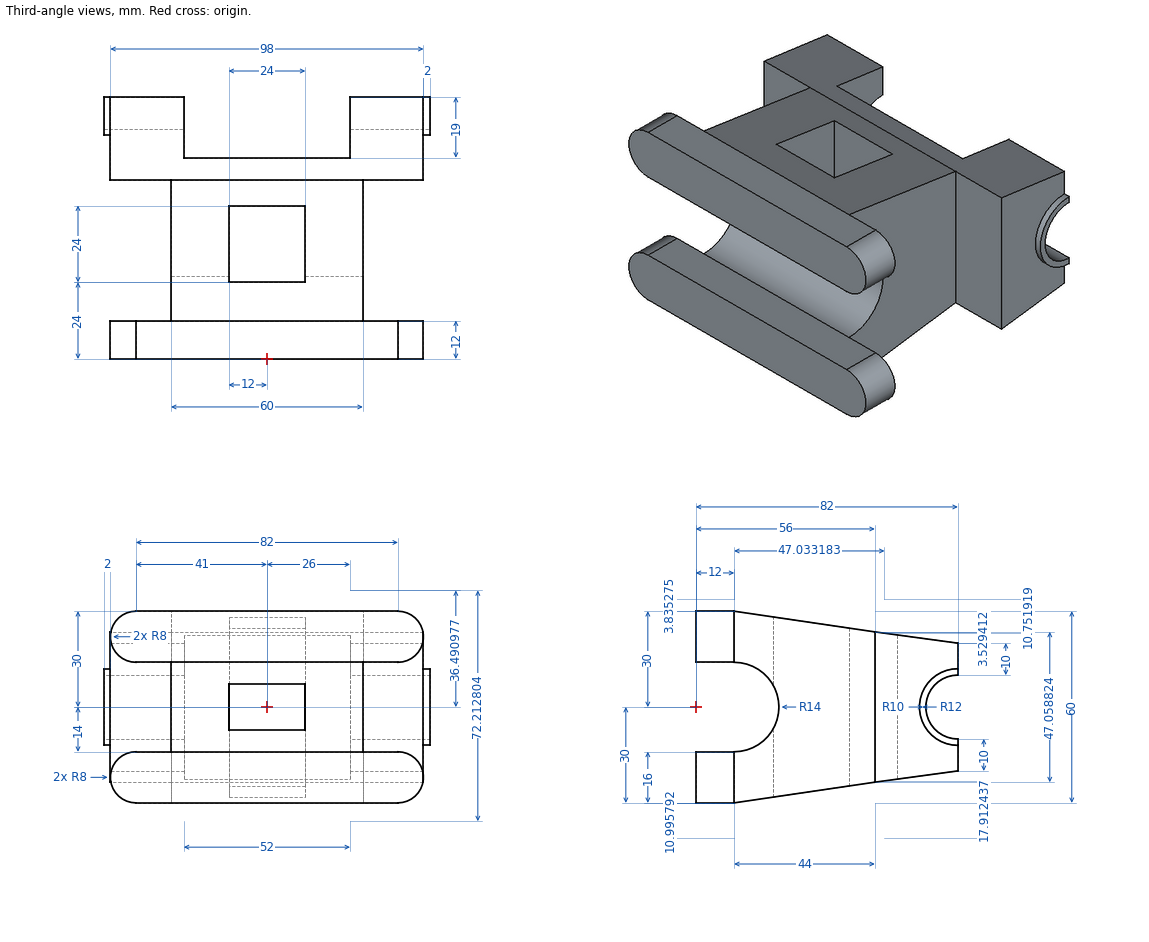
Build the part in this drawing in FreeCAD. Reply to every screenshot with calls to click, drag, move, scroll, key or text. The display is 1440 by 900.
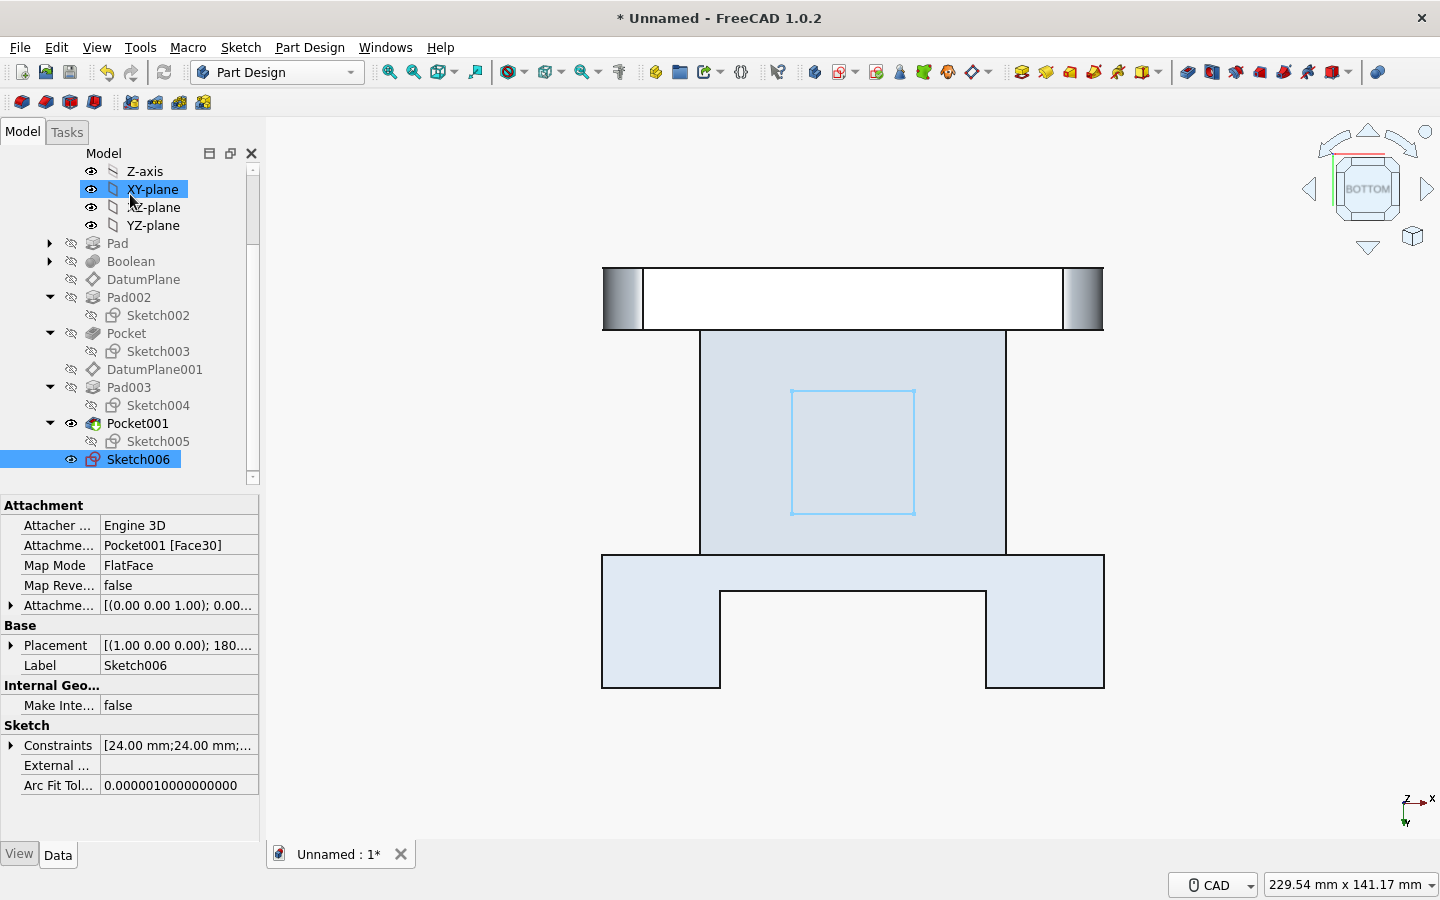
click(1188, 72)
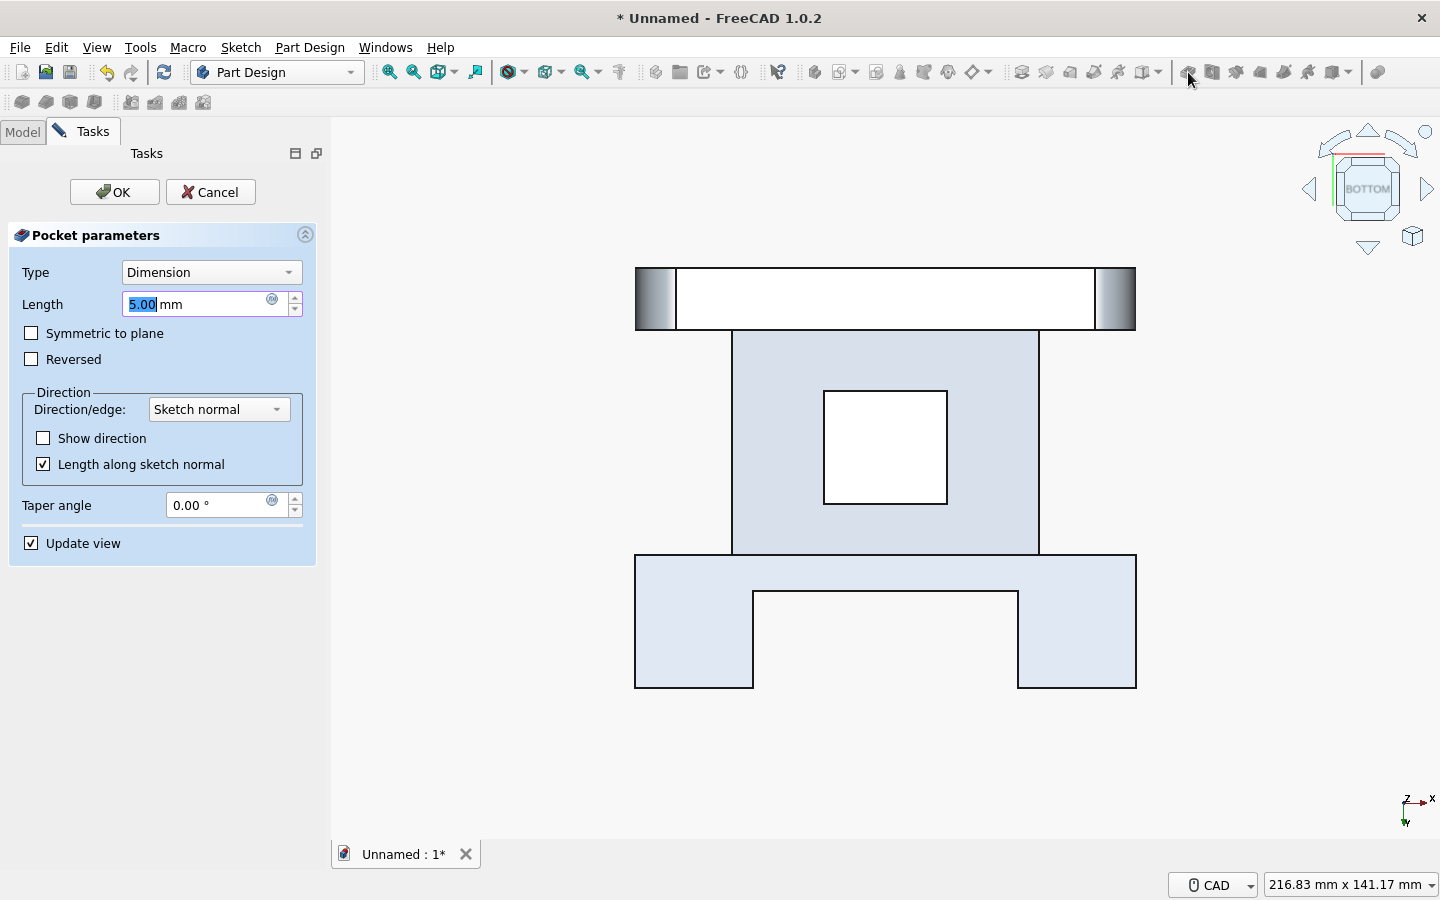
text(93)
key(Tab)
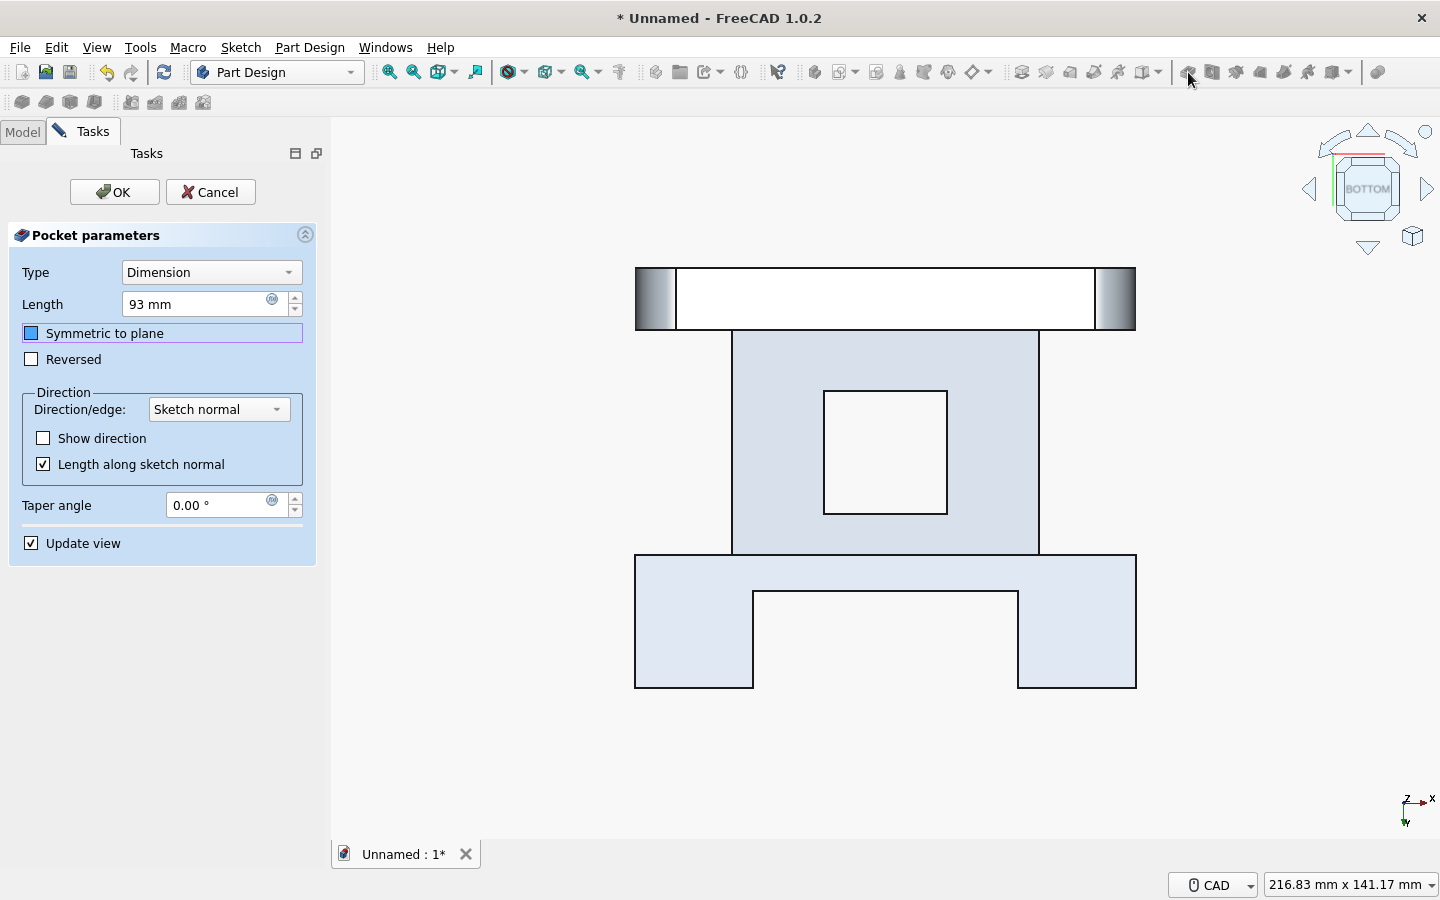
click(115, 192)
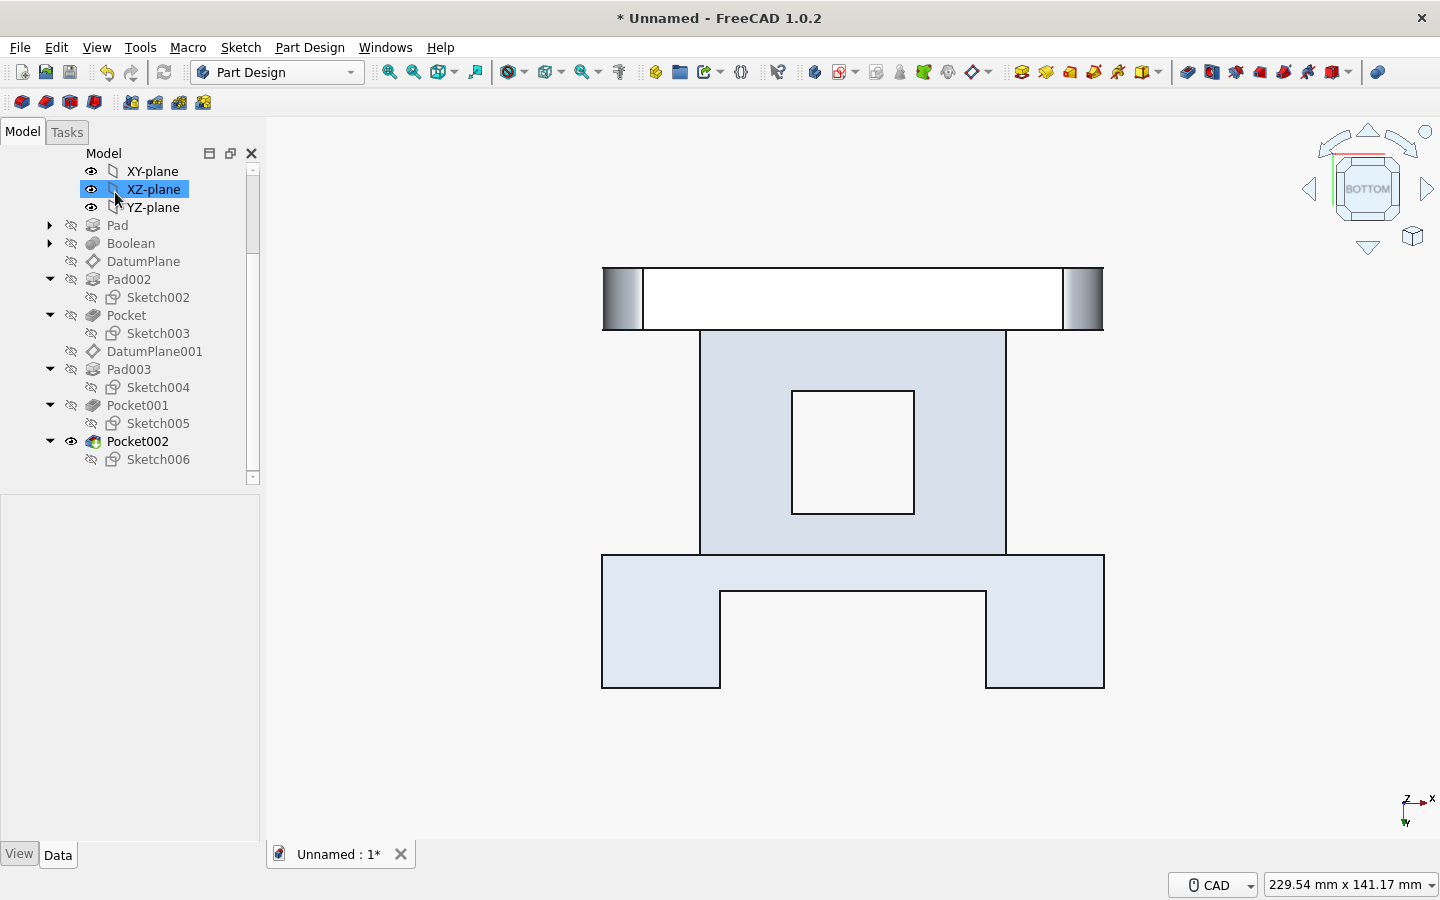
scroll(160, 311, down, 3)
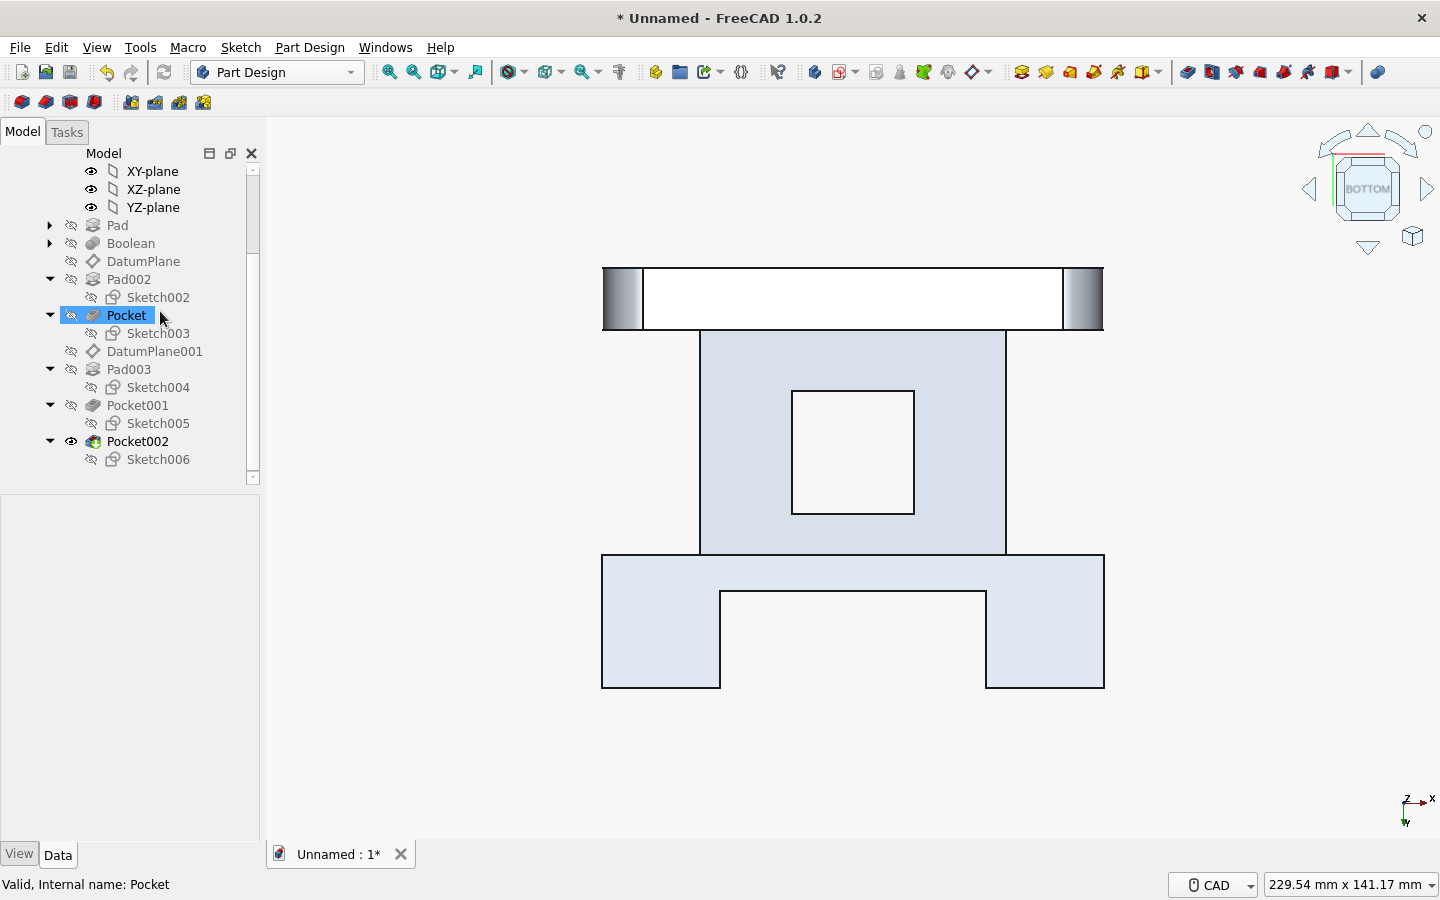
scroll(160, 311, up, 15)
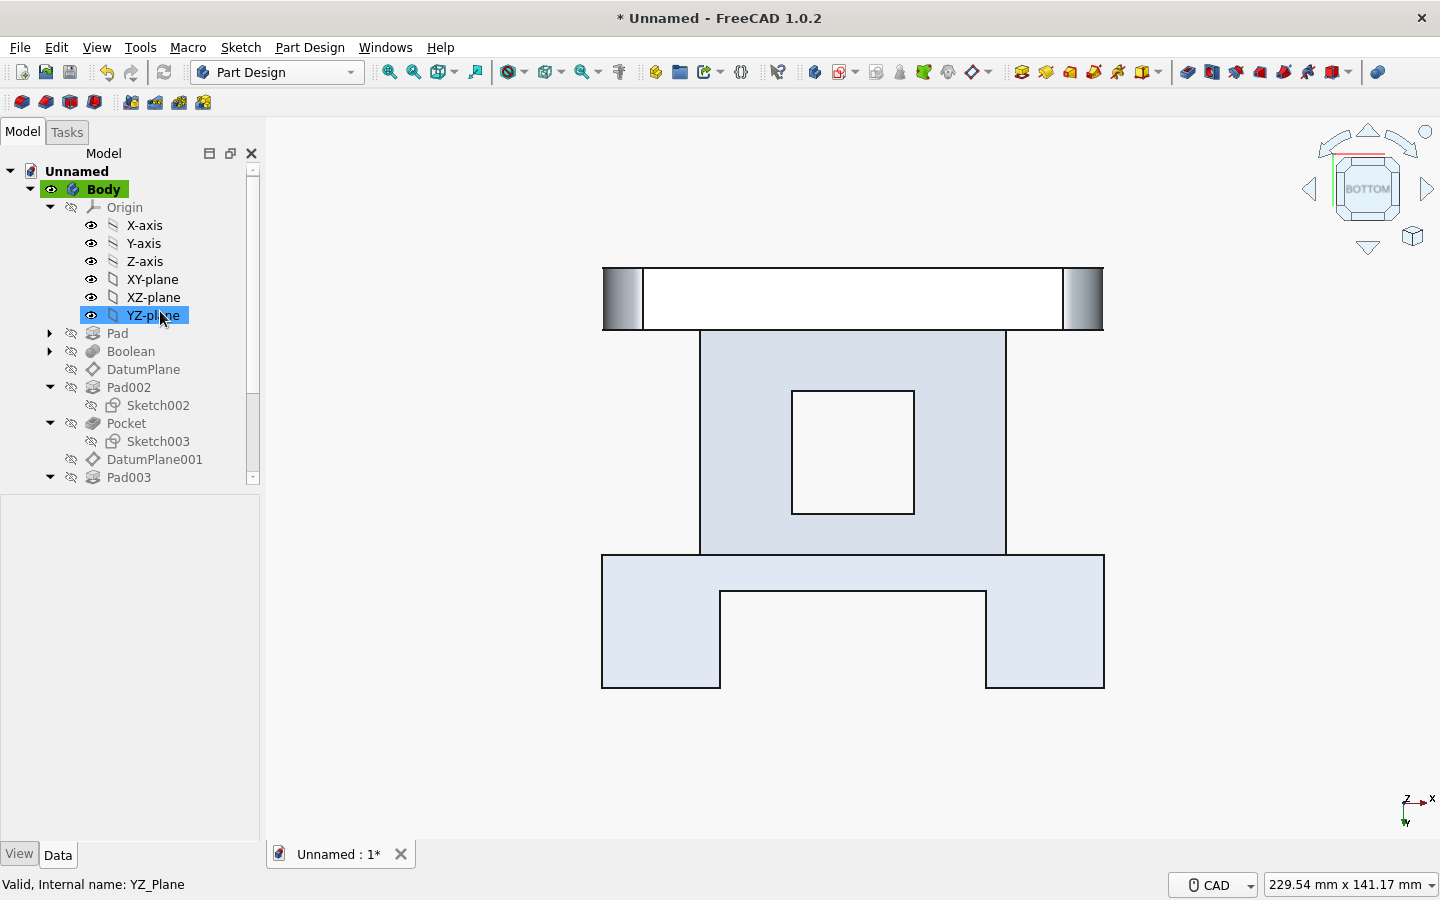
click(136, 315)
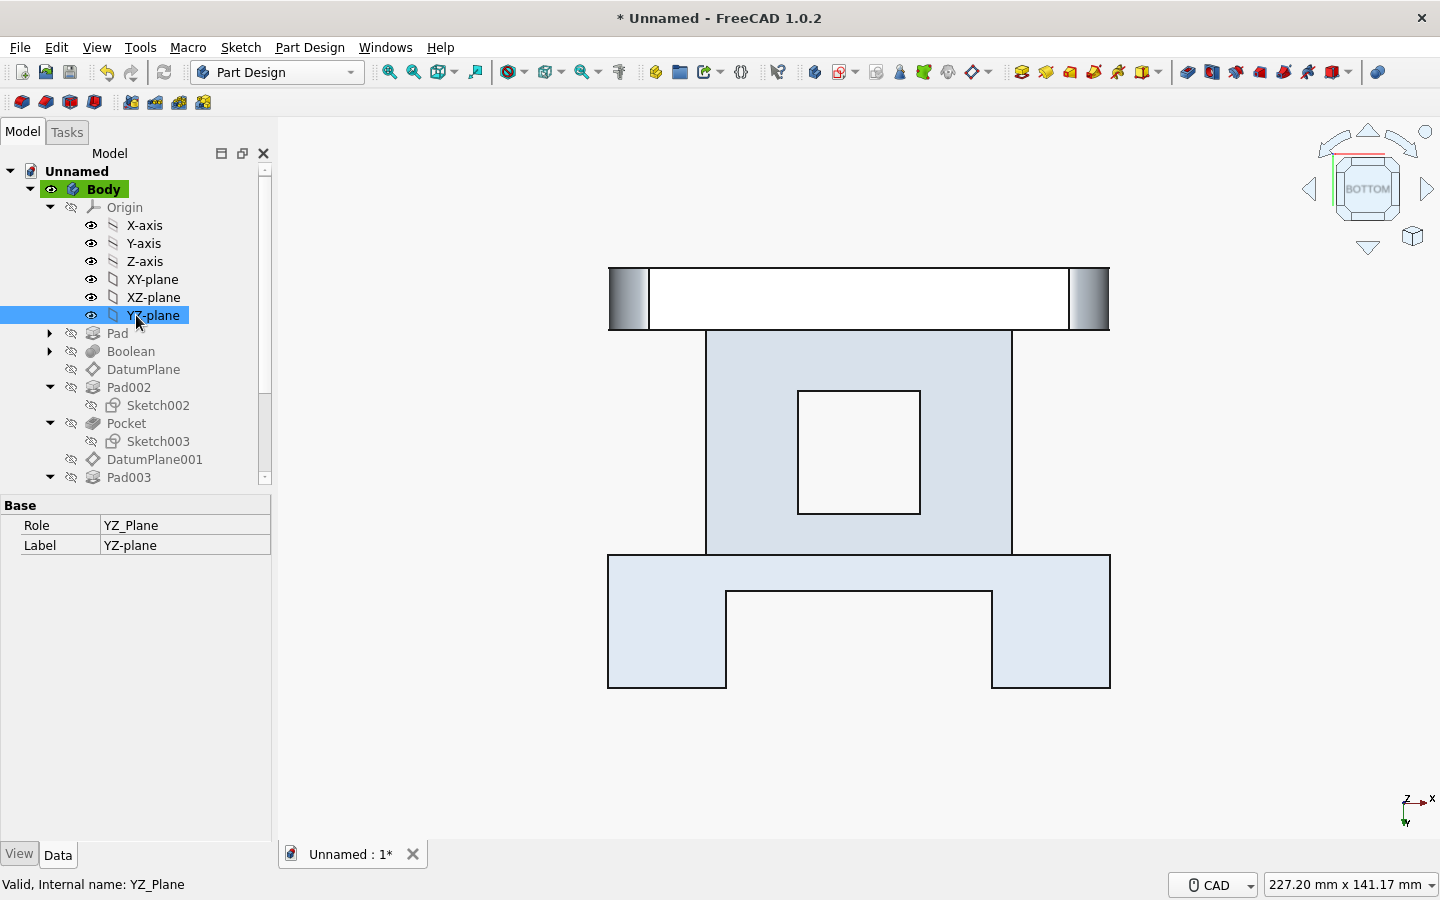
click(972, 72)